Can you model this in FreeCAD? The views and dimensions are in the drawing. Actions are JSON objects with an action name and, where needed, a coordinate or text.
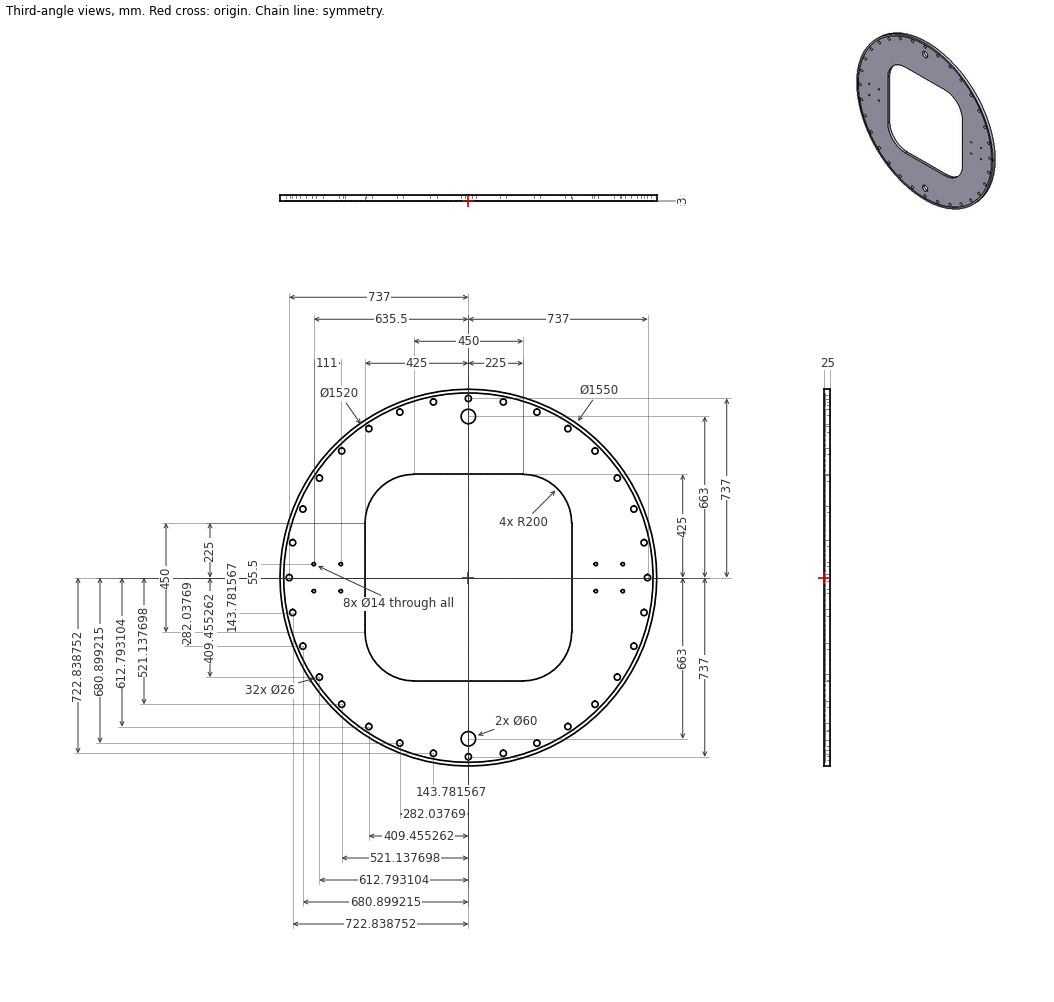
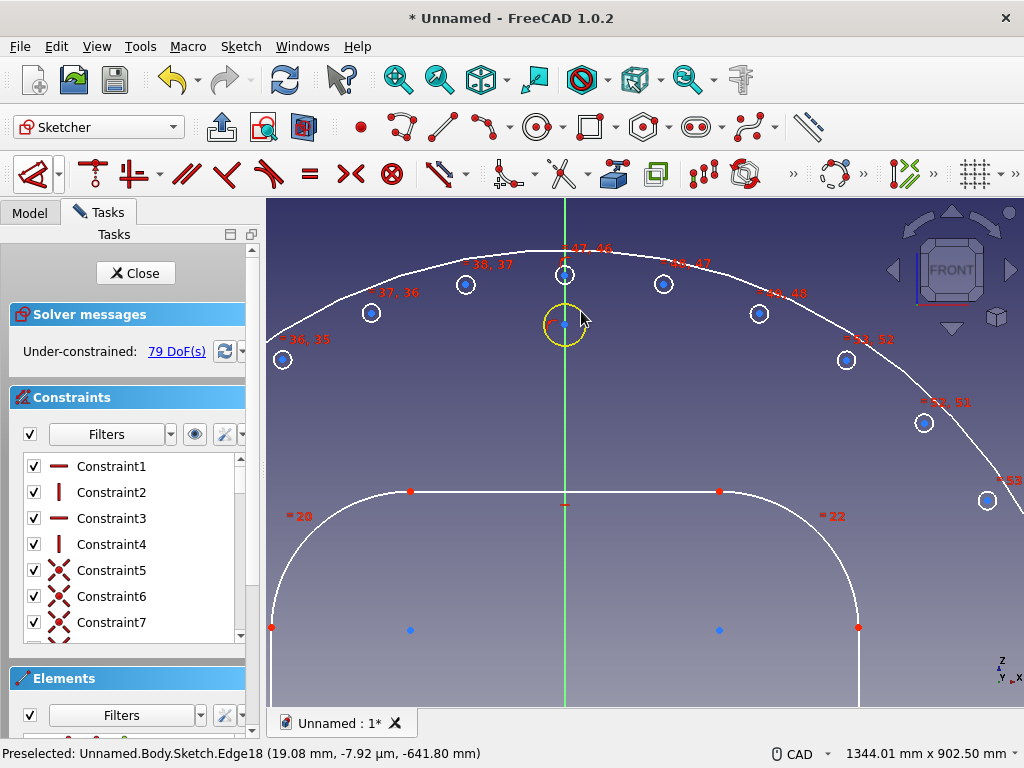
{"action": "left_click", "coordinate": [580, 310]}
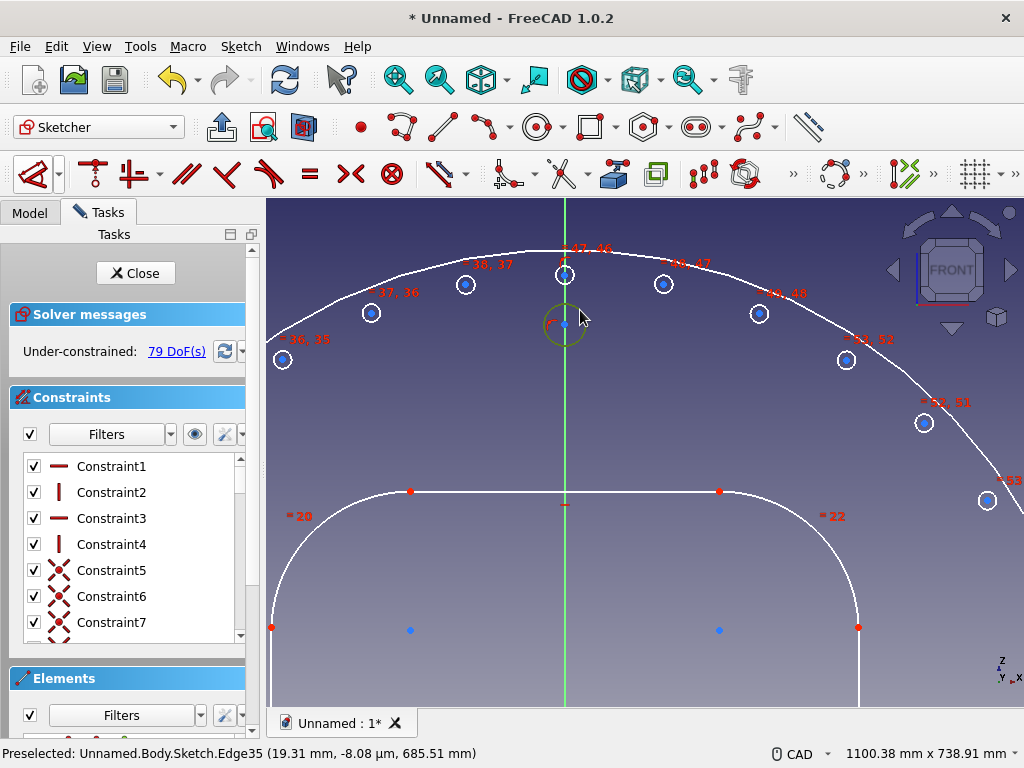
{"action": "left_click", "coordinate": [310, 174]}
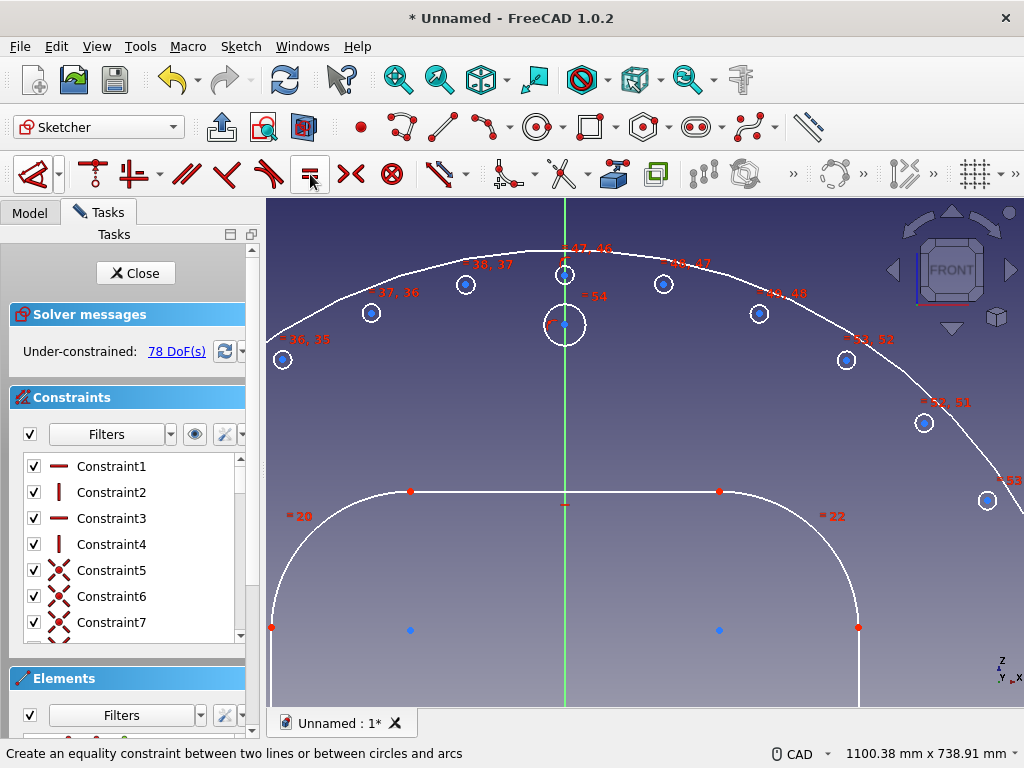
{"action": "scroll", "coordinate": [581, 311], "scroll_direction": "down", "scroll_amount": 6}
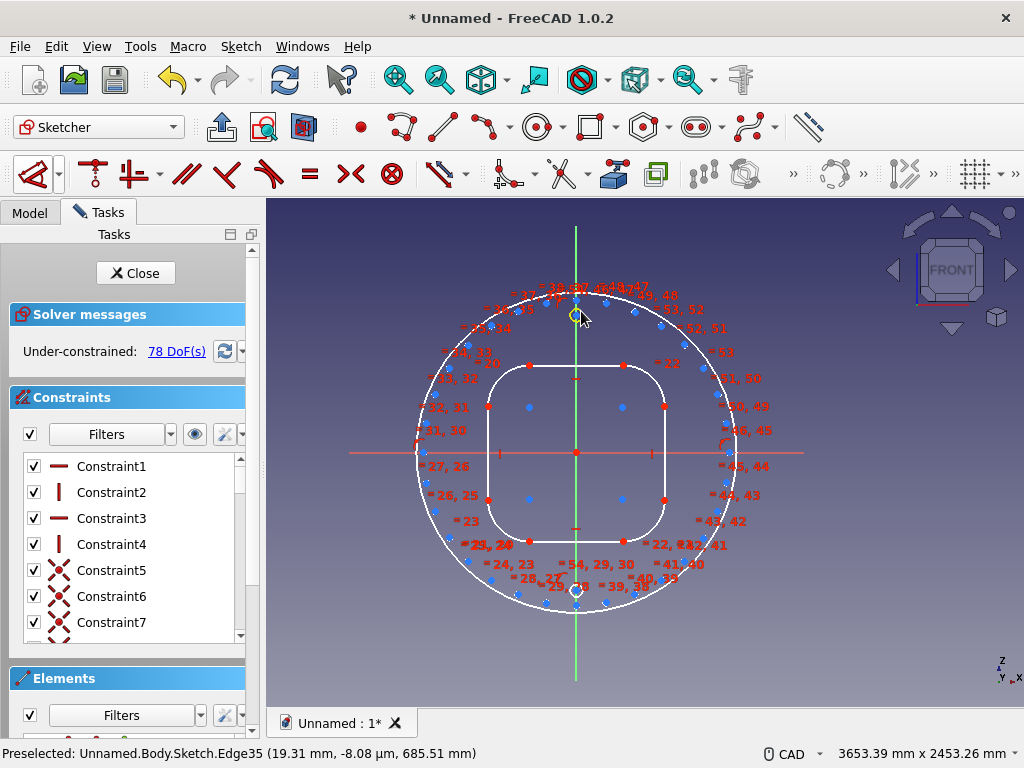
{"action": "left_click", "coordinate": [426, 483]}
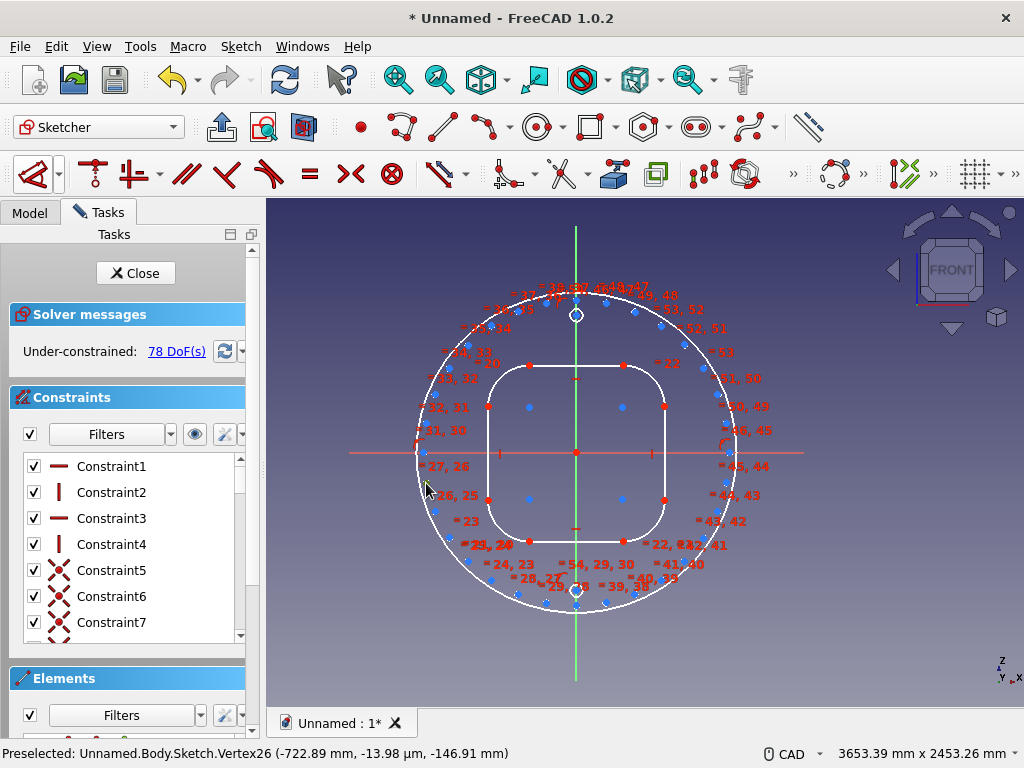
{"action": "left_click", "coordinate": [426, 423]}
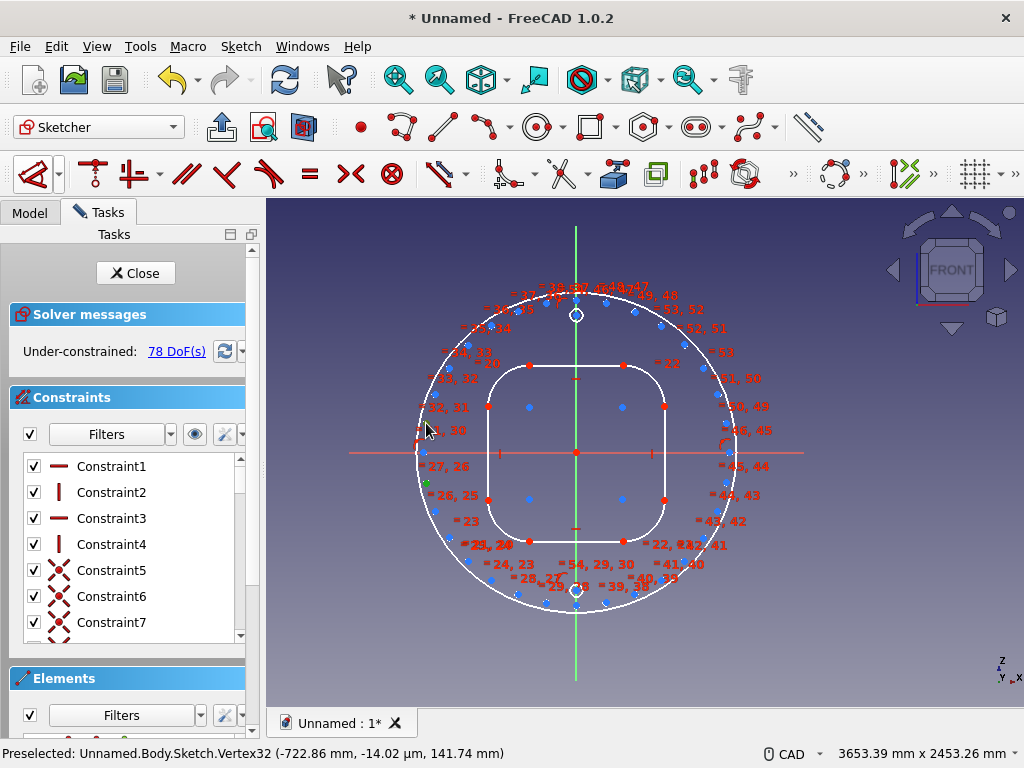
{"action": "left_click", "coordinate": [375, 453]}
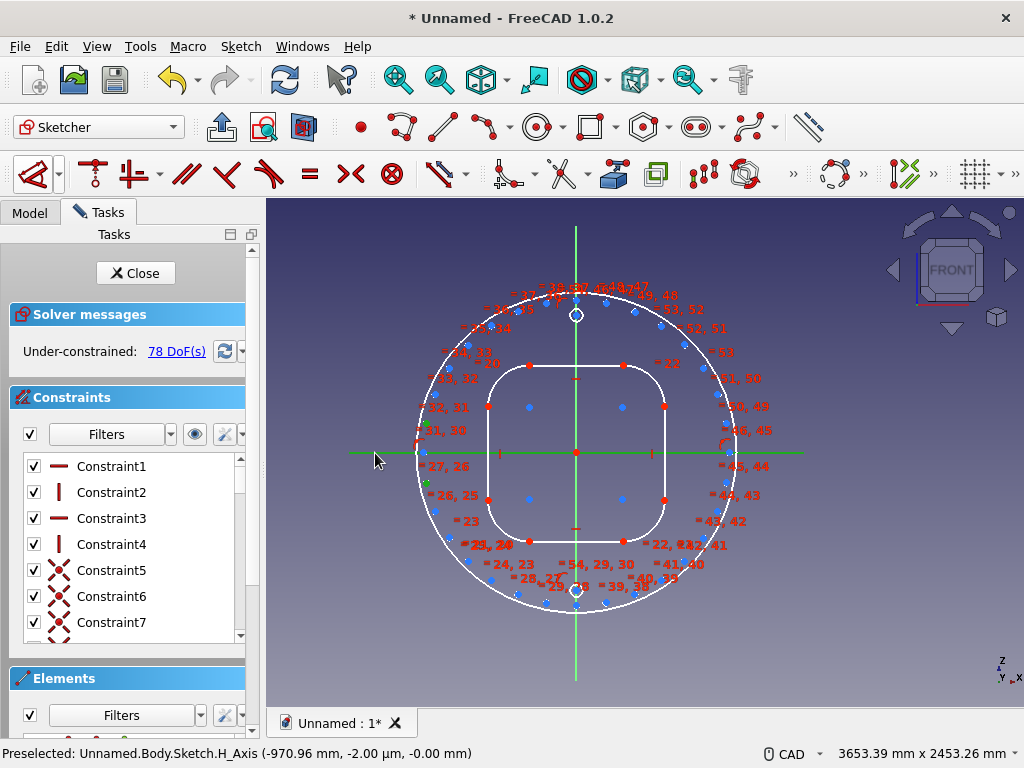
{"action": "left_click", "coordinate": [351, 174]}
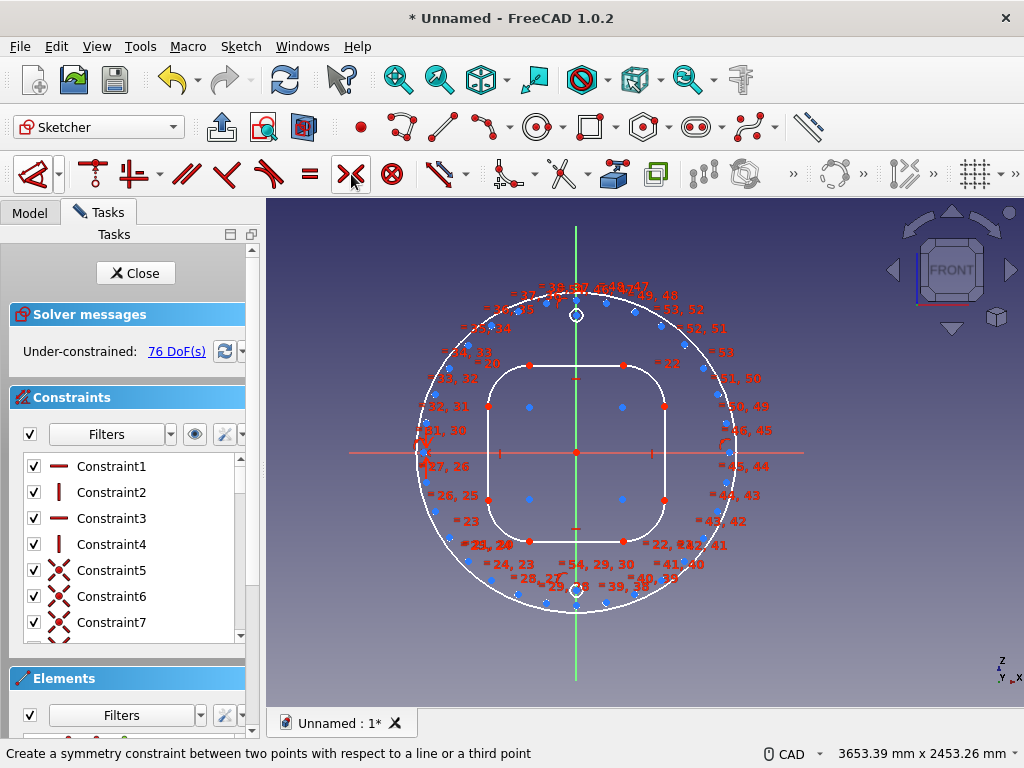
{"action": "left_click", "coordinate": [435, 512]}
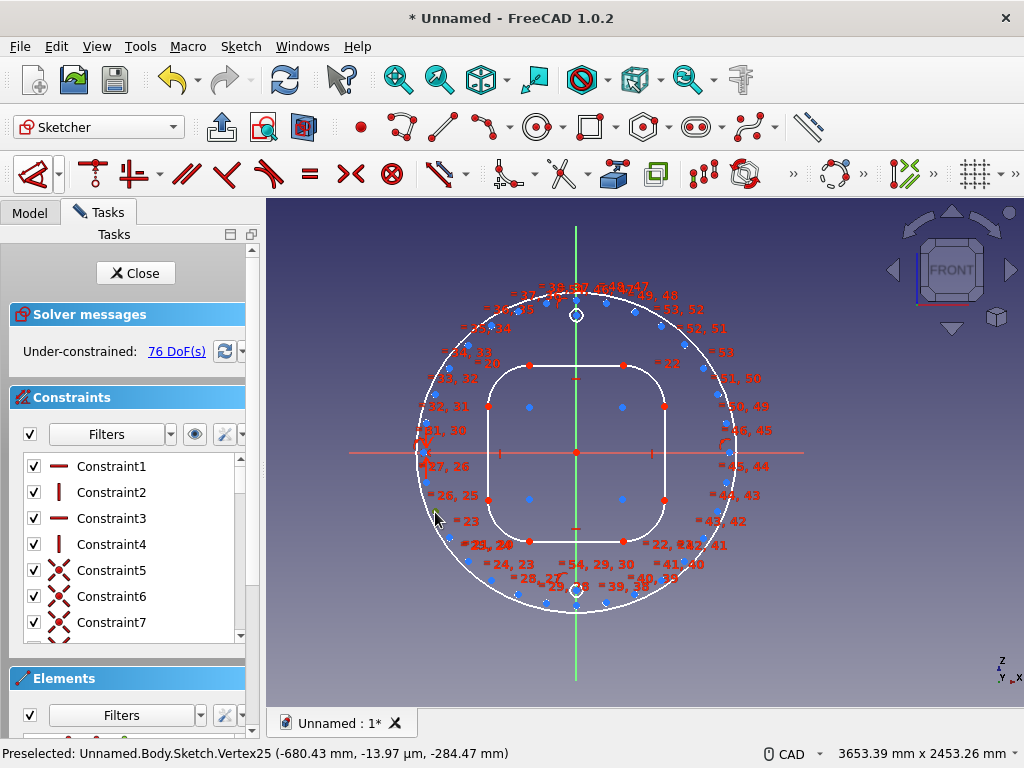
{"action": "left_click", "coordinate": [435, 395]}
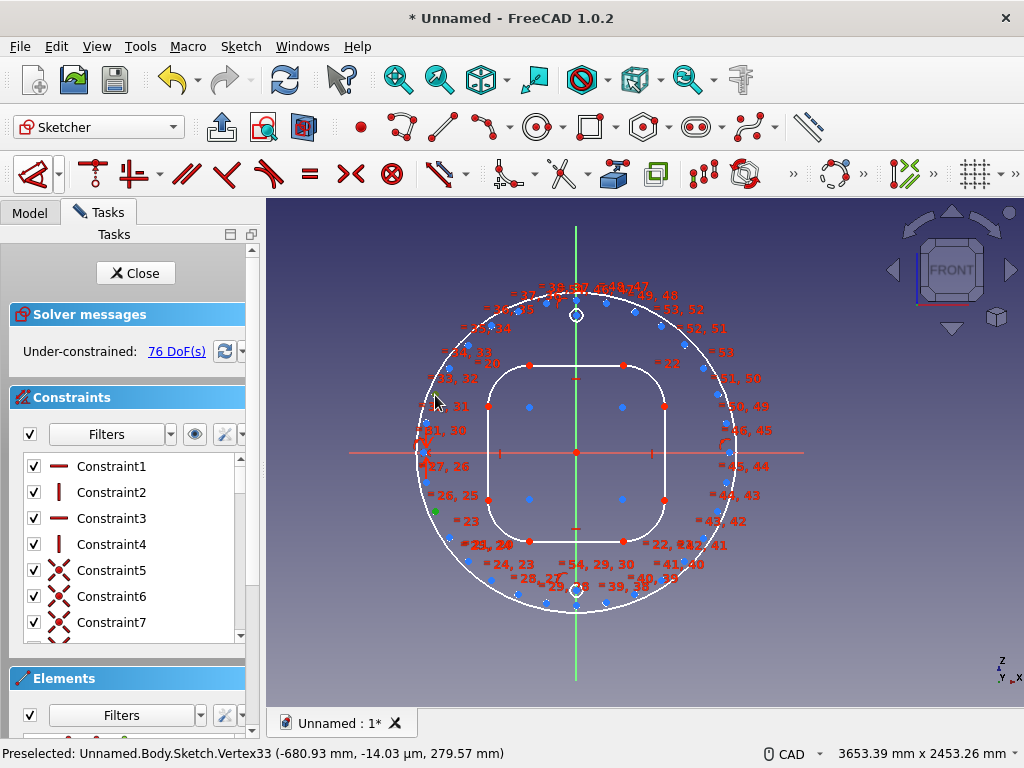
{"action": "left_click", "coordinate": [375, 453]}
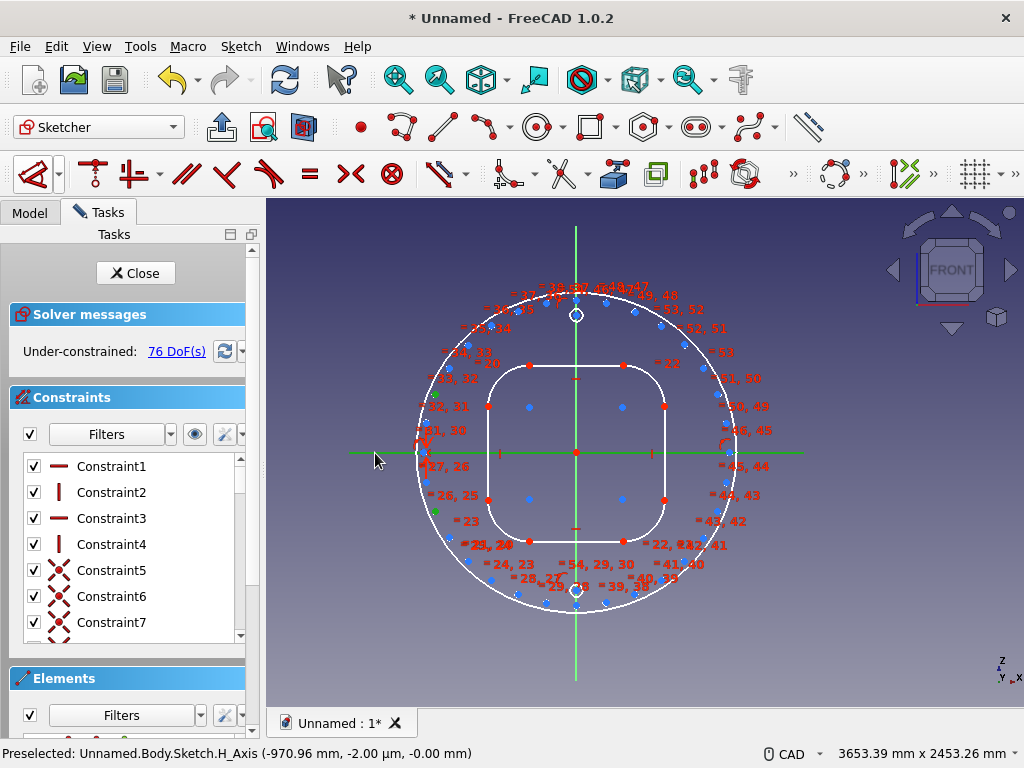
{"action": "left_click", "coordinate": [351, 174]}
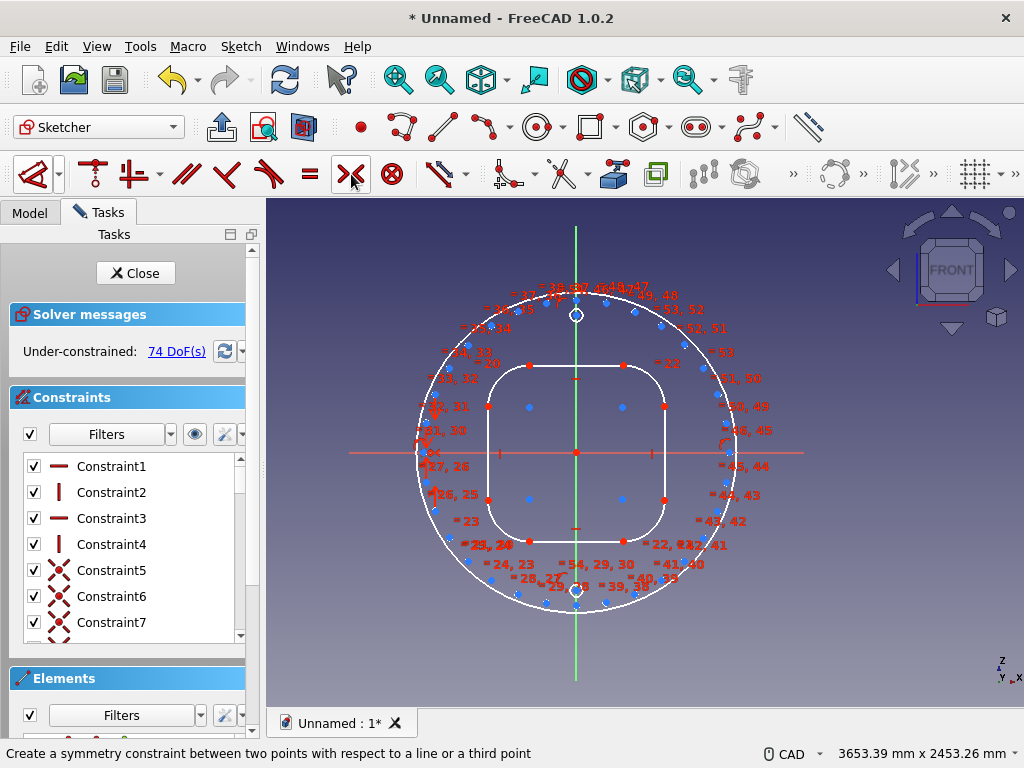
{"action": "left_click", "coordinate": [450, 538]}